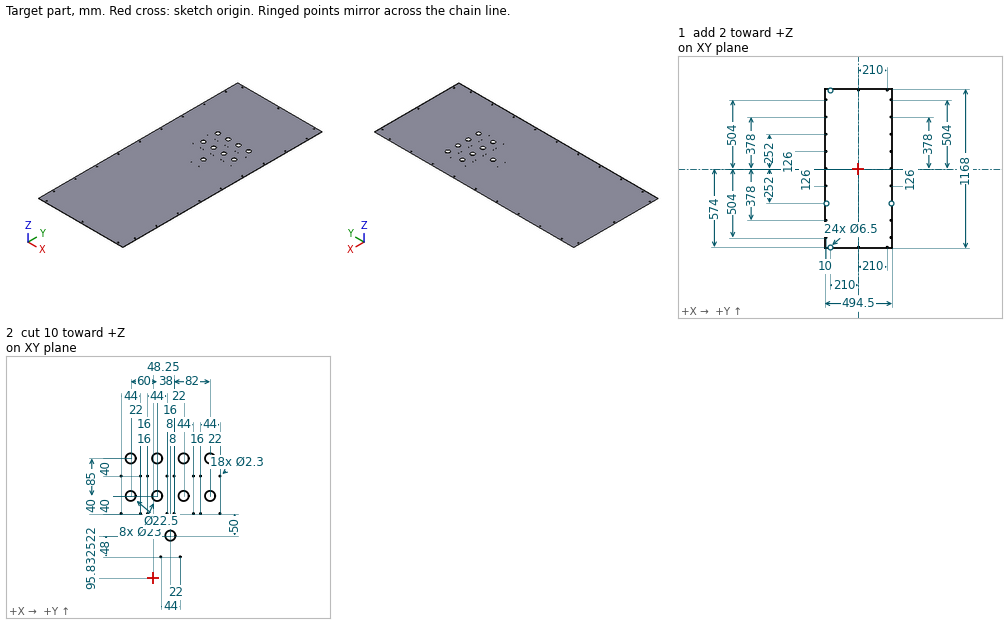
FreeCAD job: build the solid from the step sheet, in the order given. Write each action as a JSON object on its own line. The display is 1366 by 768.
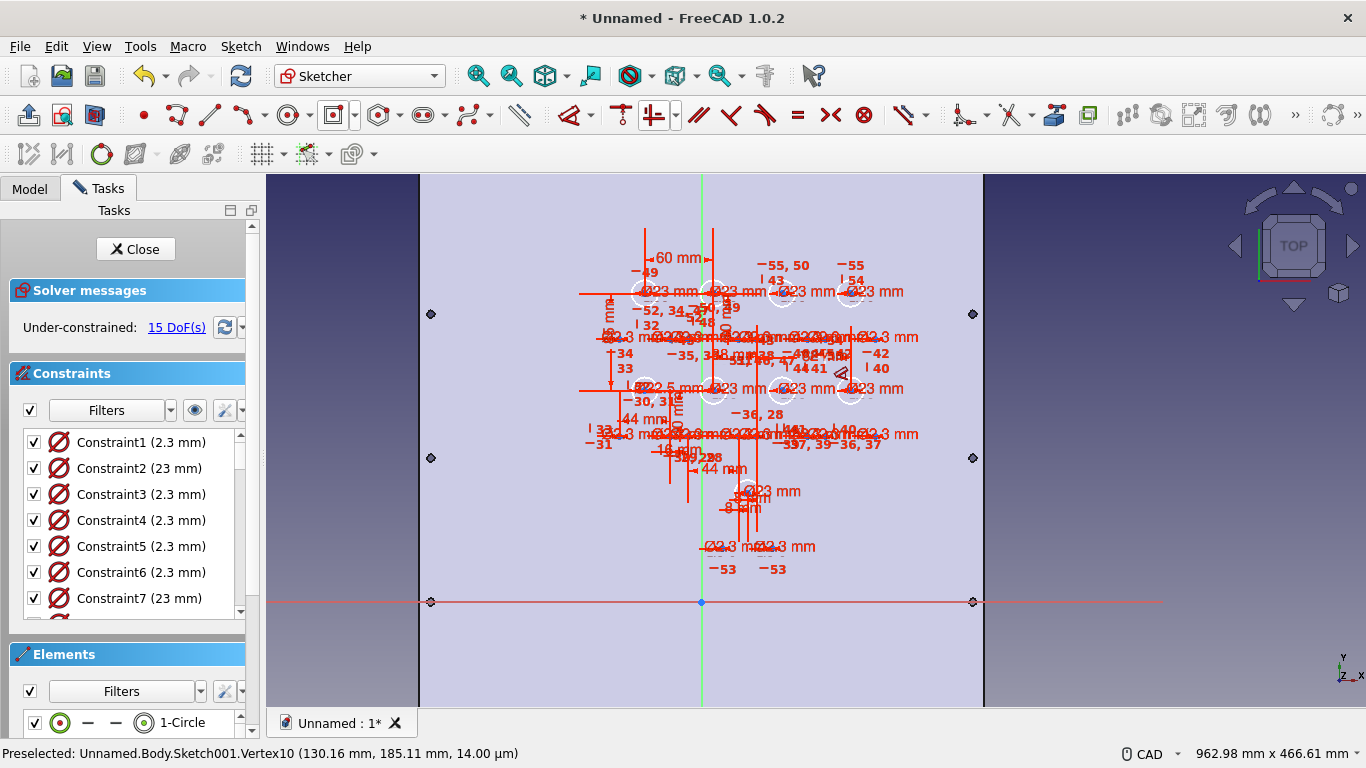
{"action": "scroll", "coordinate": [851, 391], "scroll_direction": "up", "scroll_amount": 3}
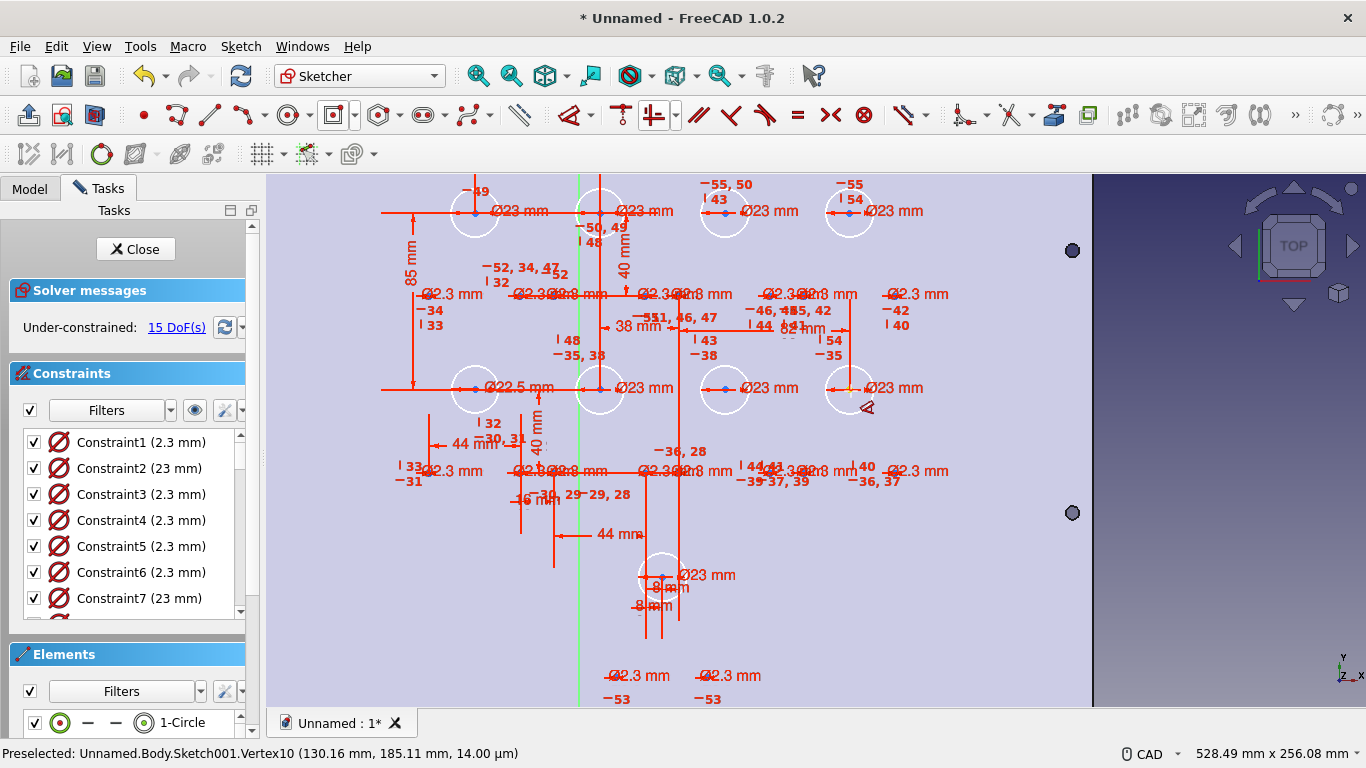
{"action": "left_click", "coordinate": [850, 390]}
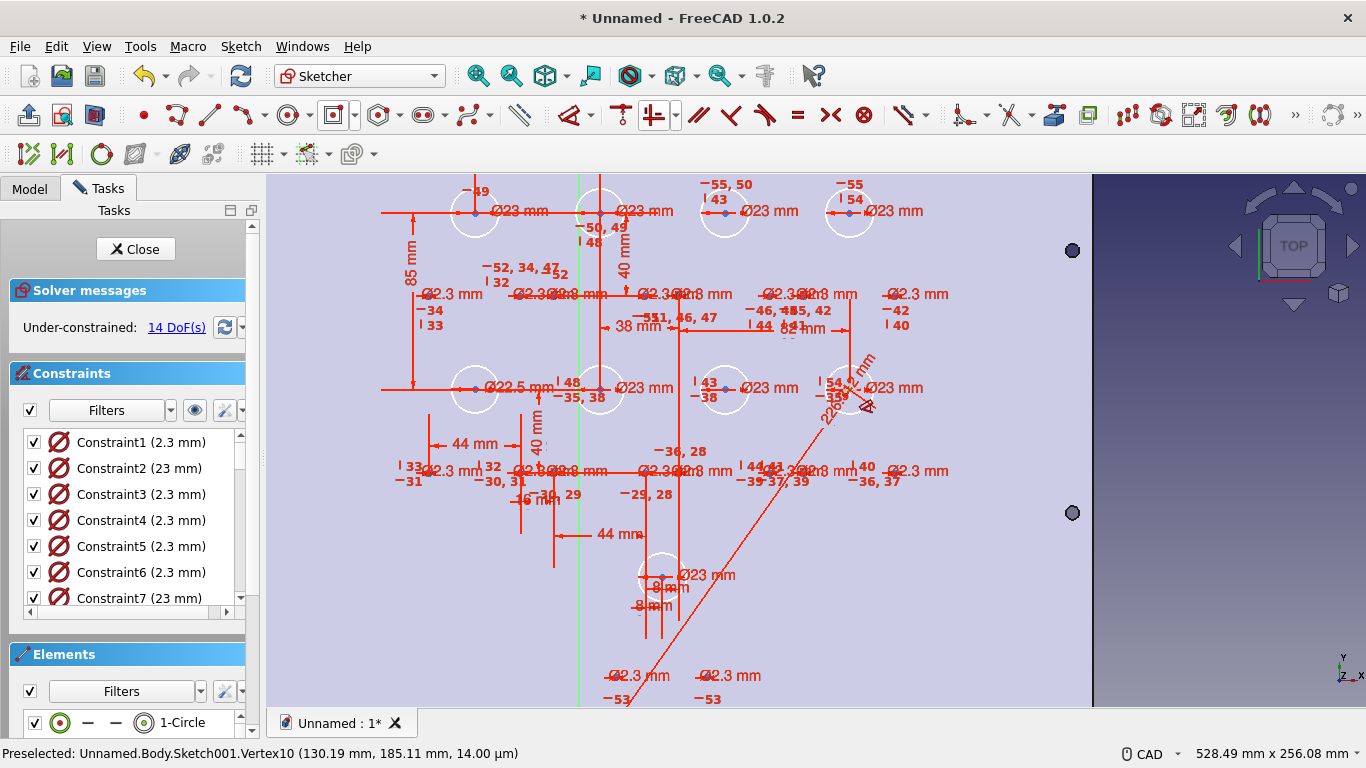
{"action": "left_click", "coordinate": [895, 473]}
{"action": "left_click", "coordinate": [872, 356]}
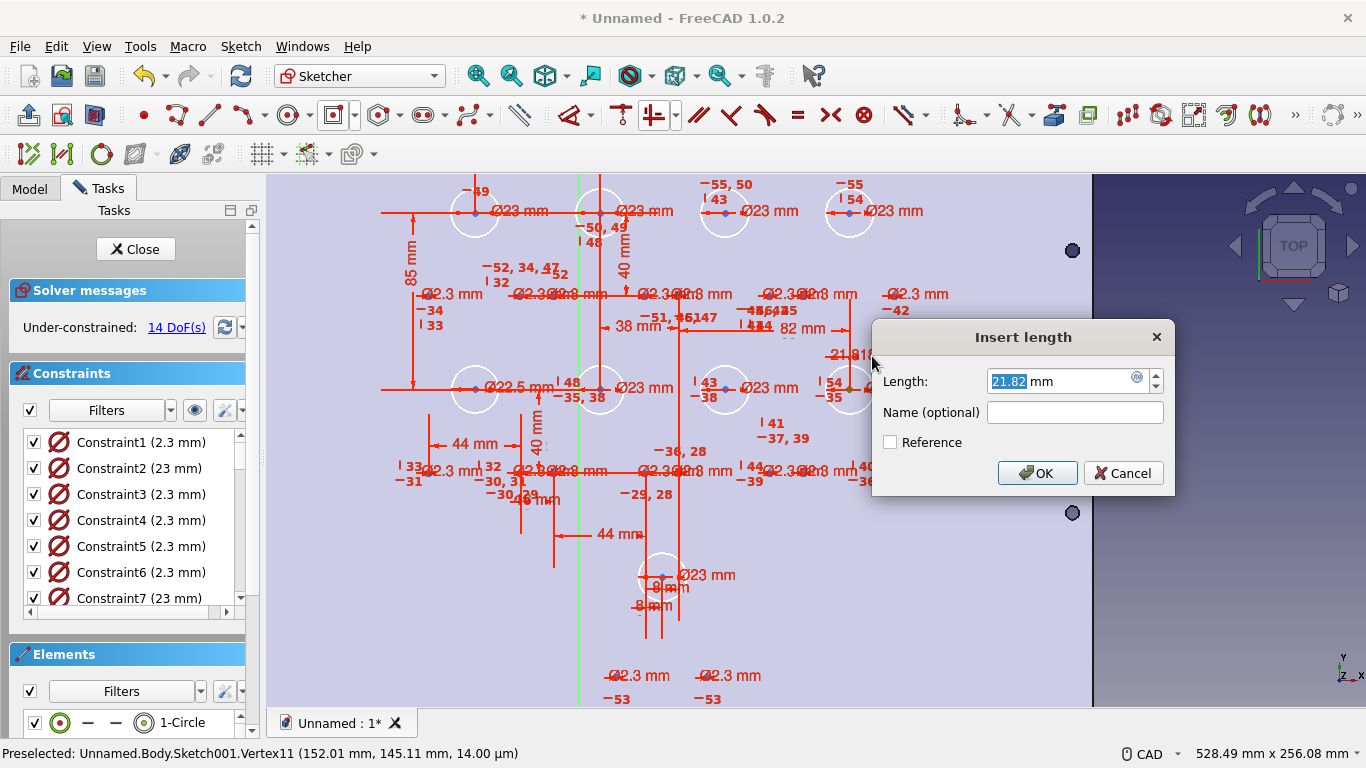
{"action": "type", "text": "22"}
{"action": "key", "text": "Return"}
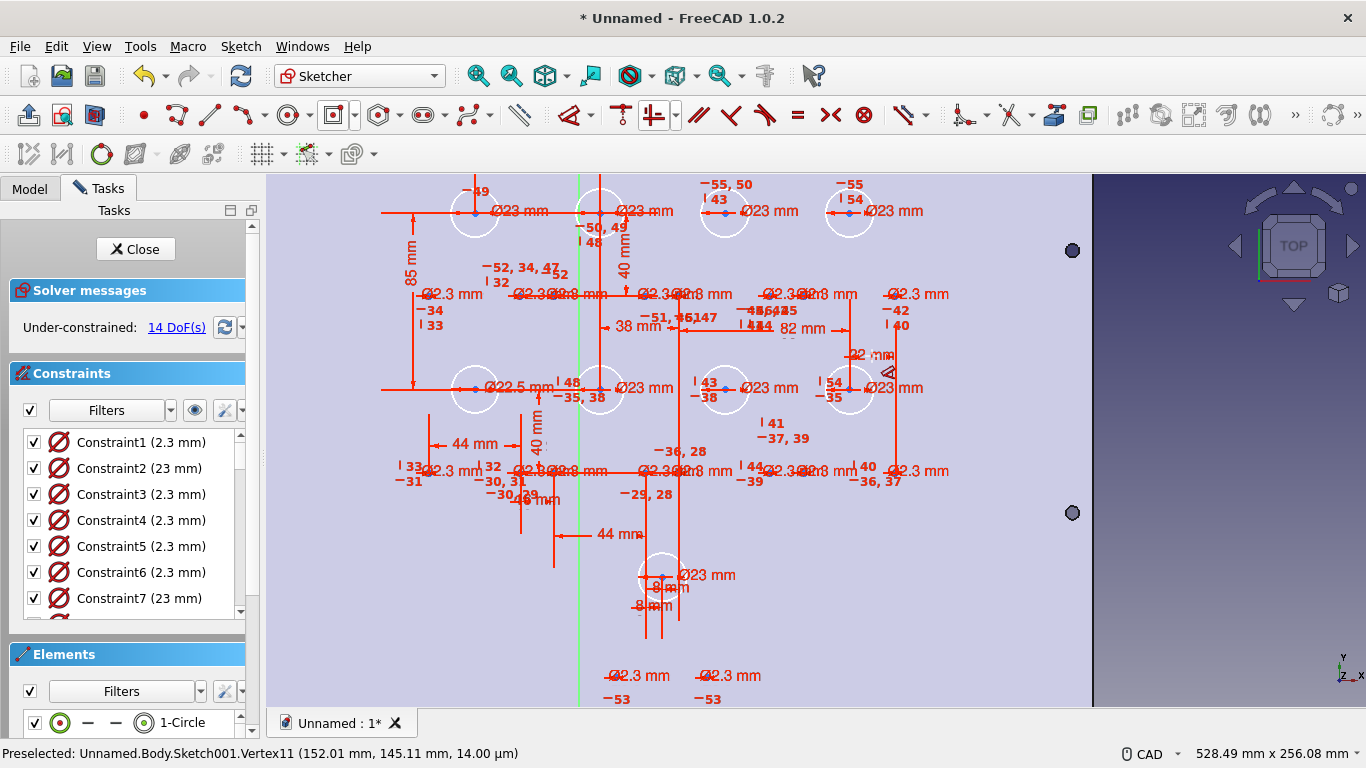
{"action": "left_click", "coordinate": [896, 473]}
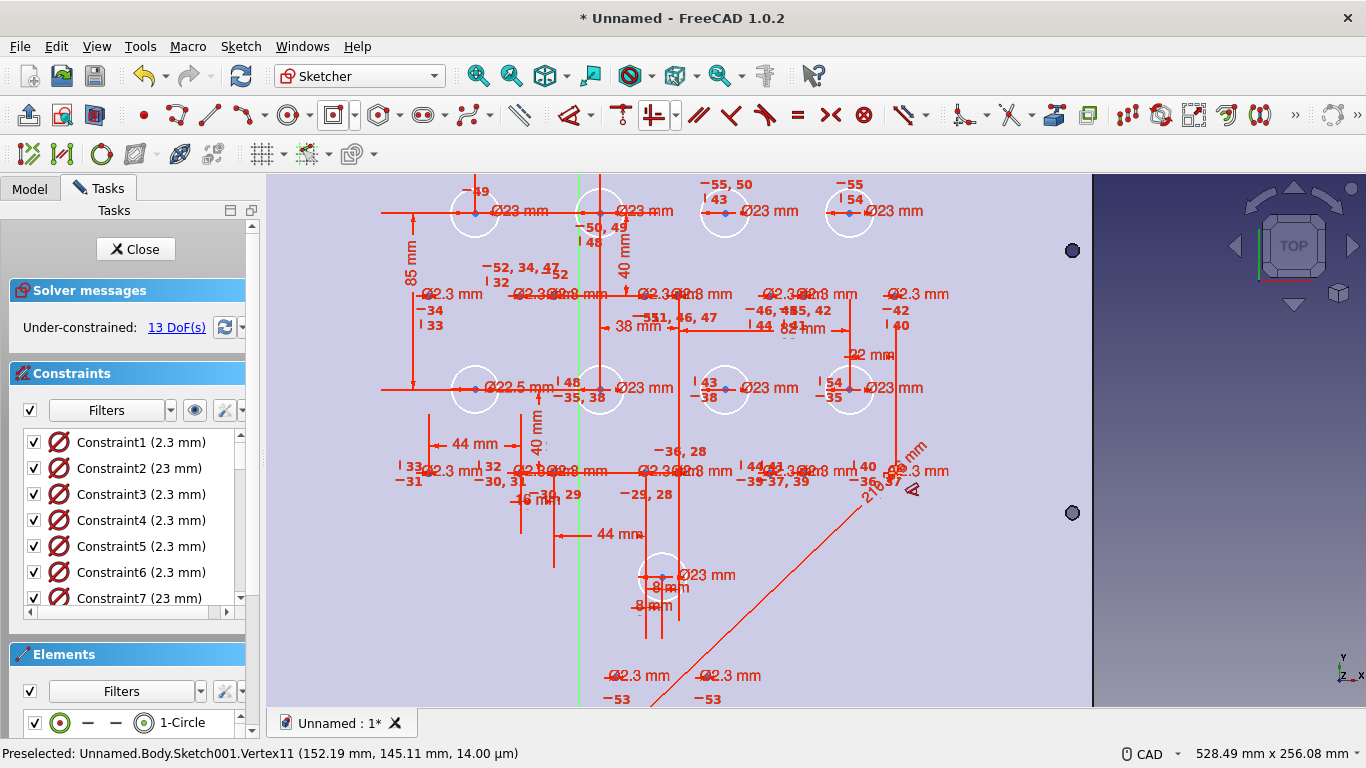
{"action": "left_click", "coordinate": [804, 473]}
{"action": "left_click", "coordinate": [850, 439]}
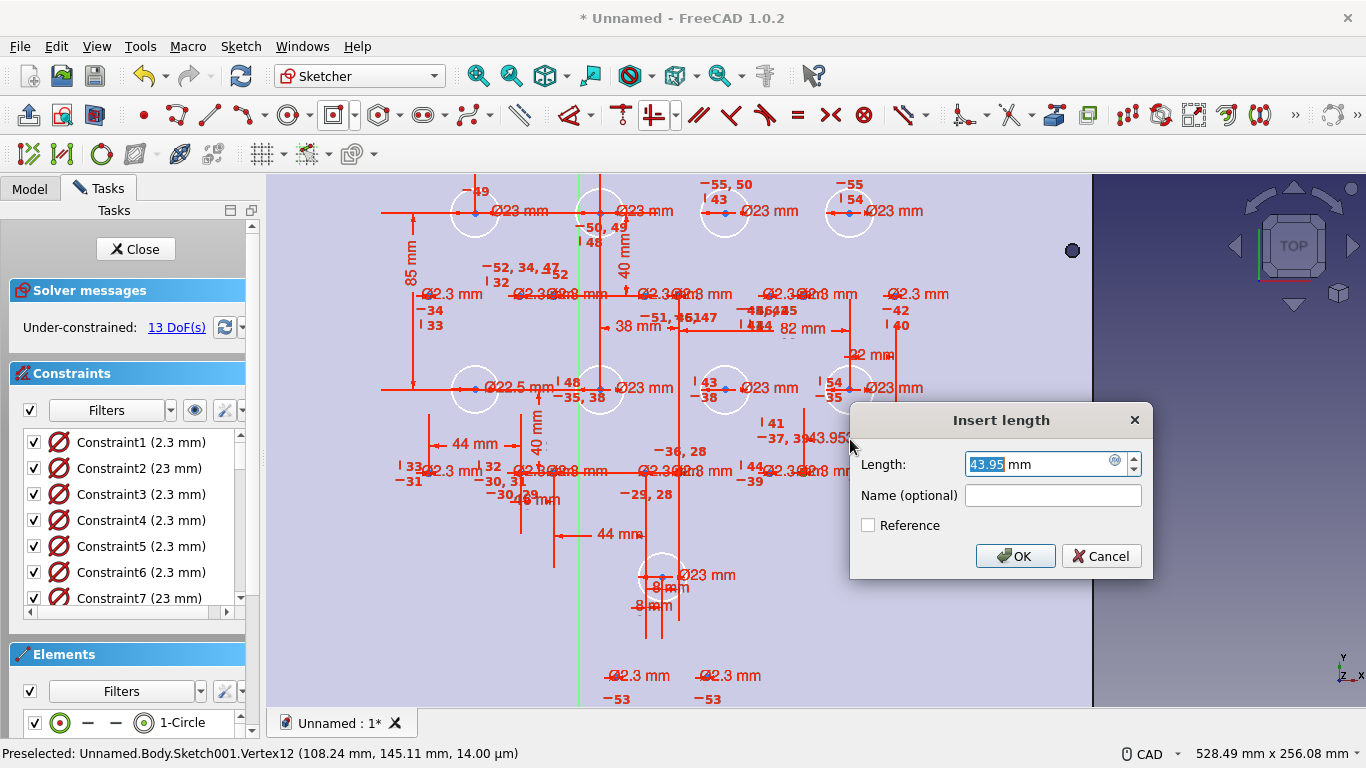
{"action": "type", "text": "44"}
{"action": "key", "text": "Return"}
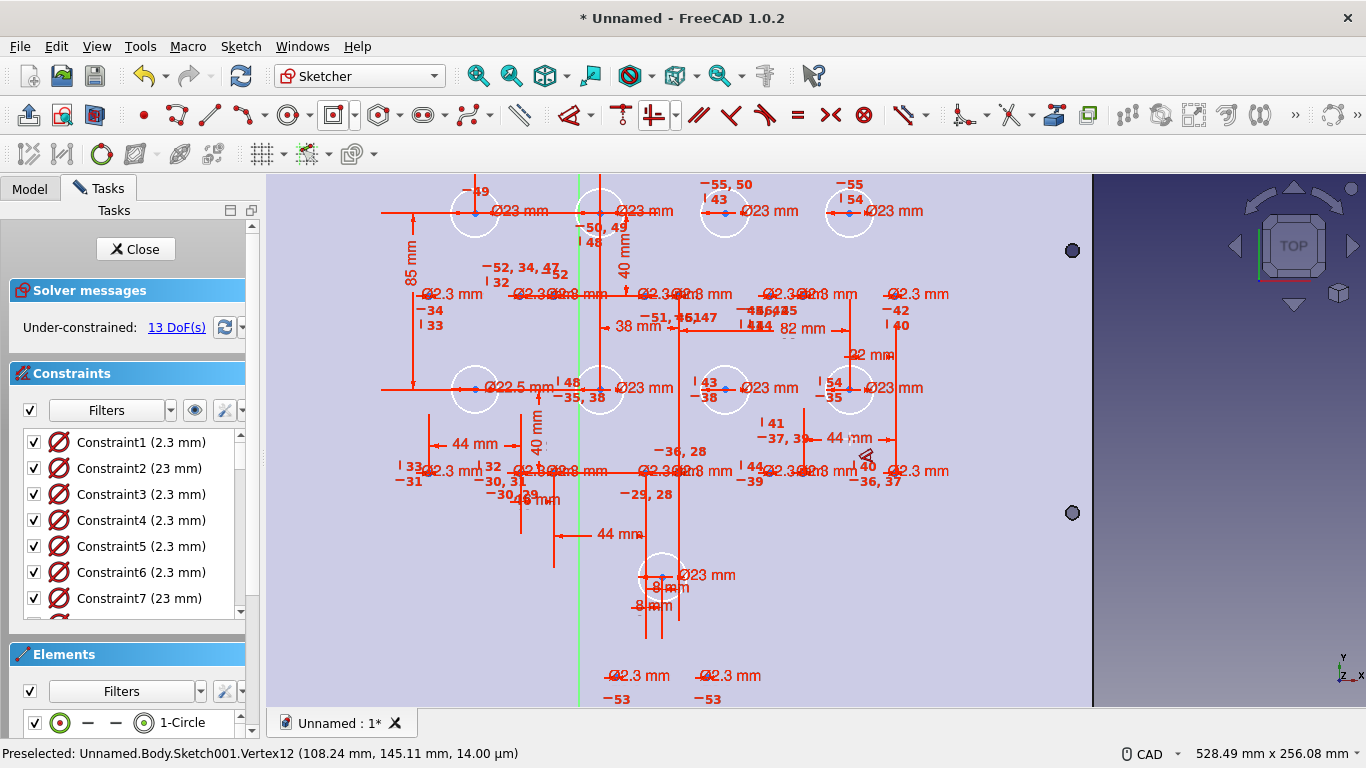
{"action": "left_click", "coordinate": [679, 473]}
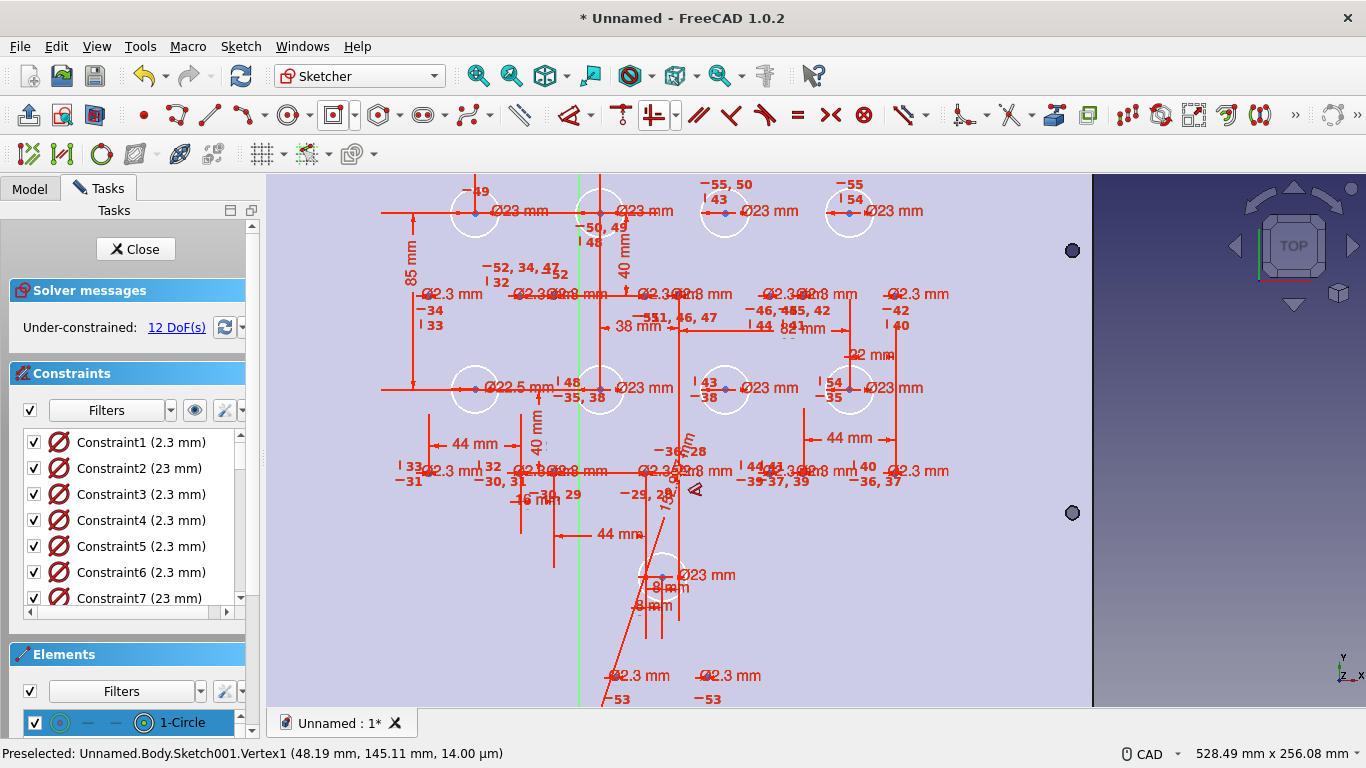
{"action": "left_click", "coordinate": [725, 390]}
{"action": "left_click", "coordinate": [702, 356]}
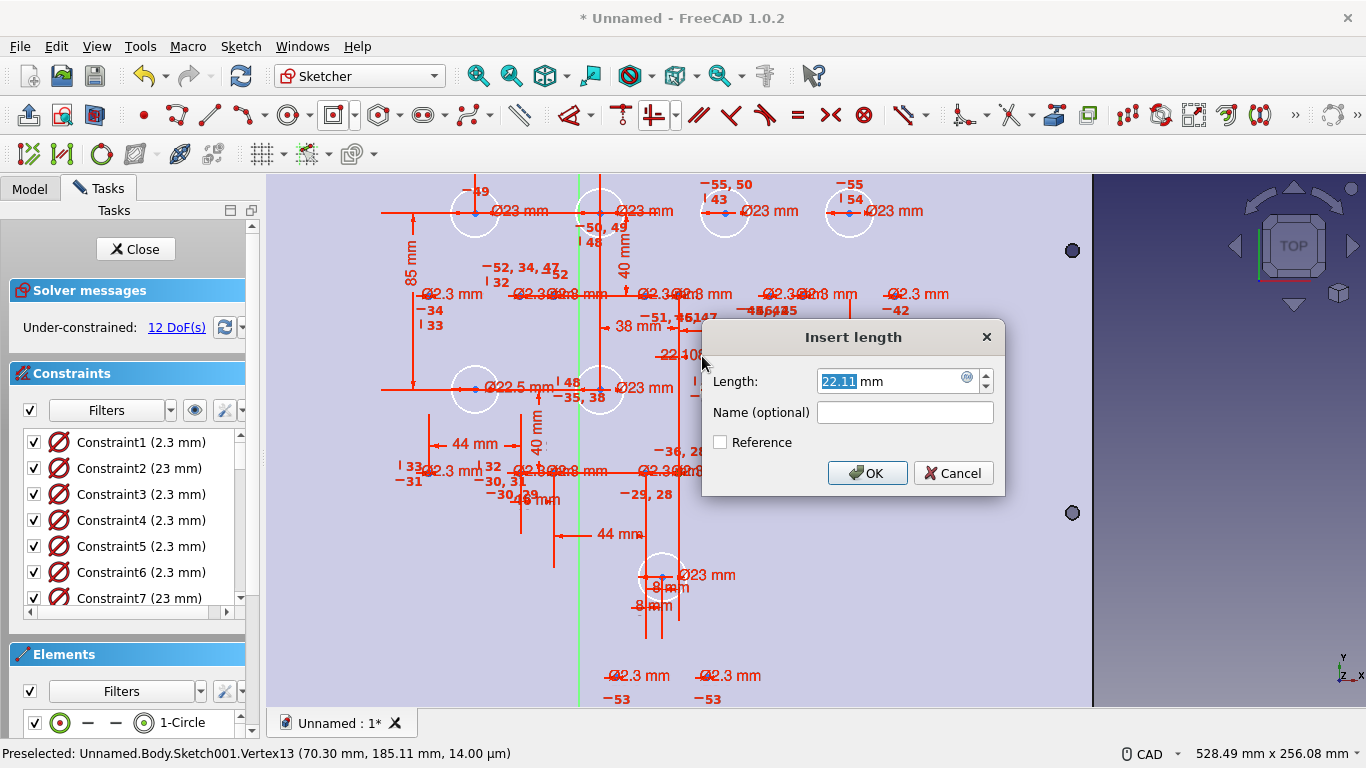
{"action": "type", "text": "22"}
{"action": "key", "text": "Return"}